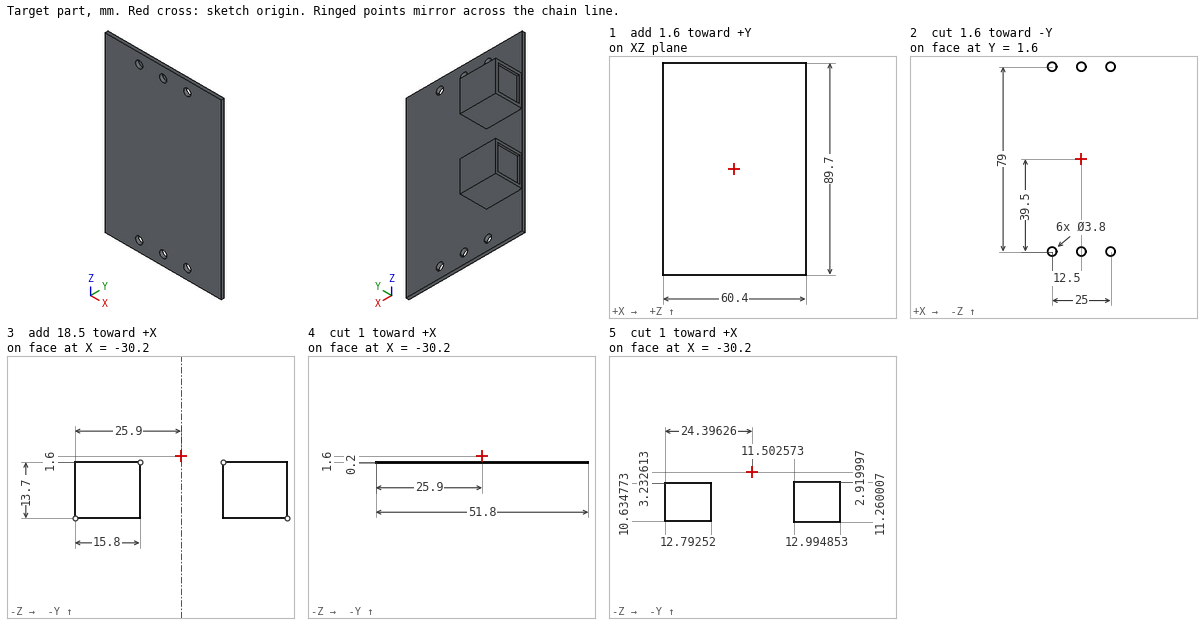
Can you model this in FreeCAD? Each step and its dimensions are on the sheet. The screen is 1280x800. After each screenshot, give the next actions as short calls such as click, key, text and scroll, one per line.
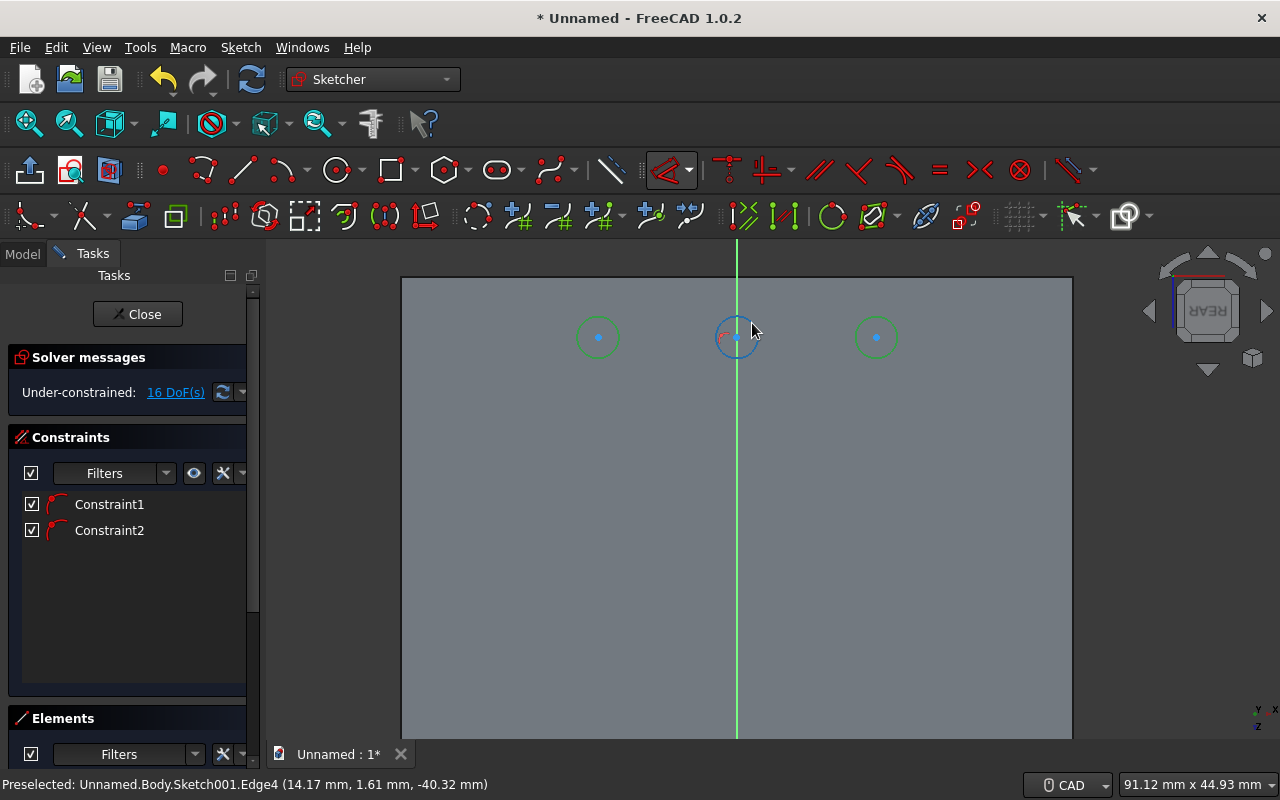
click(752, 323)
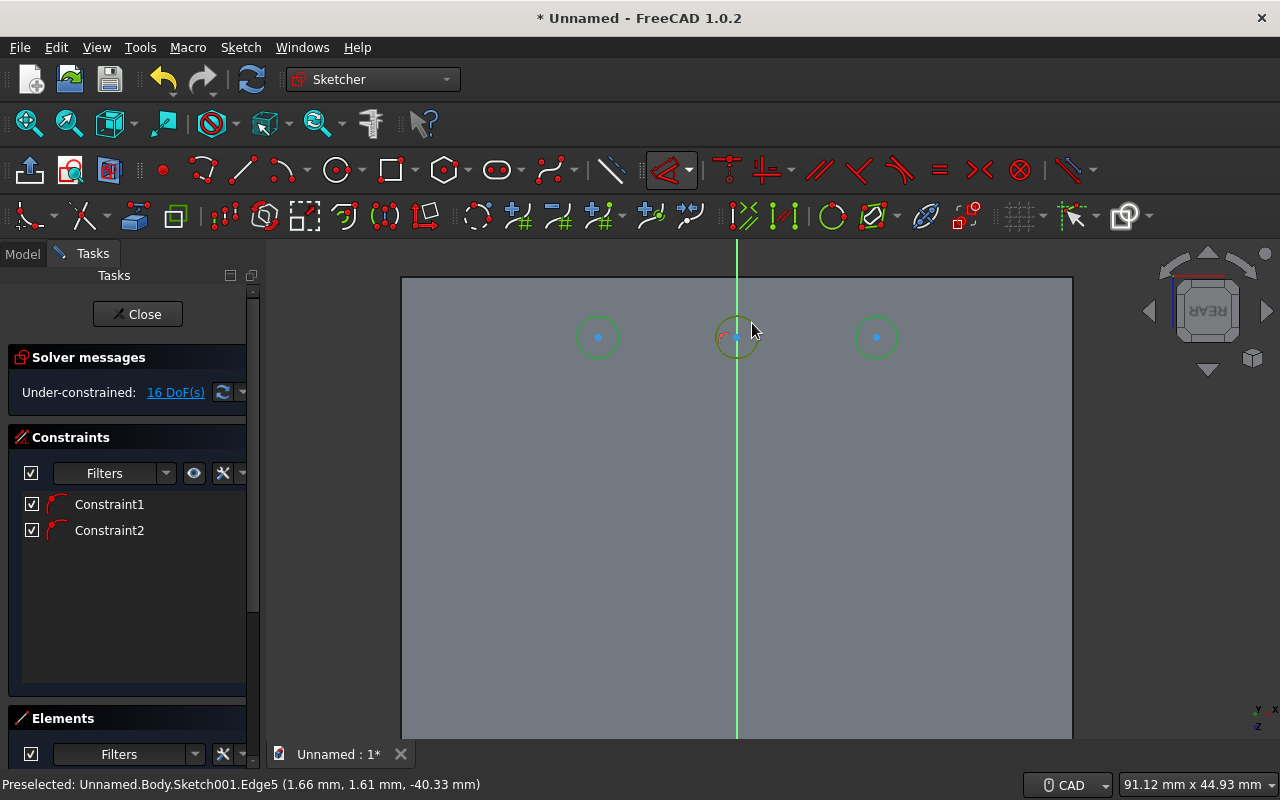
scroll(686, 322, down, 5)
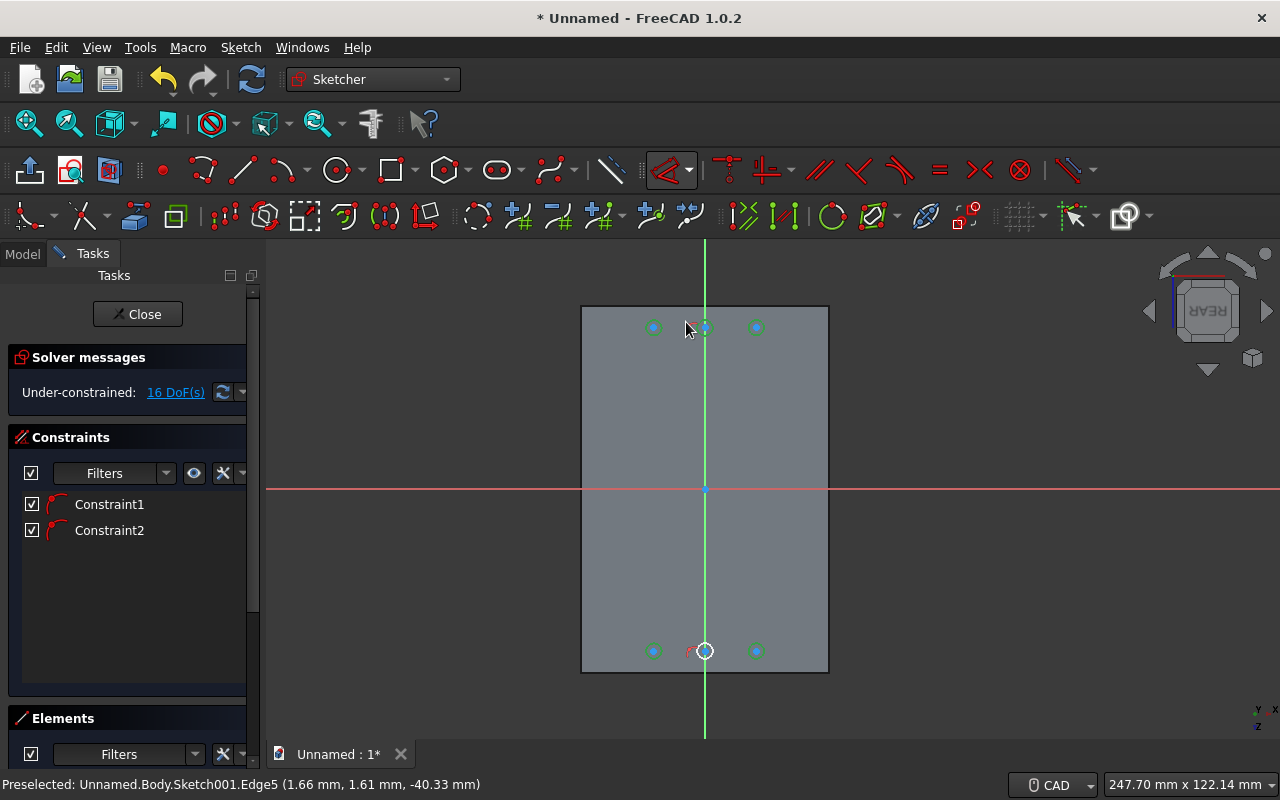
scroll(711, 645, up, 5)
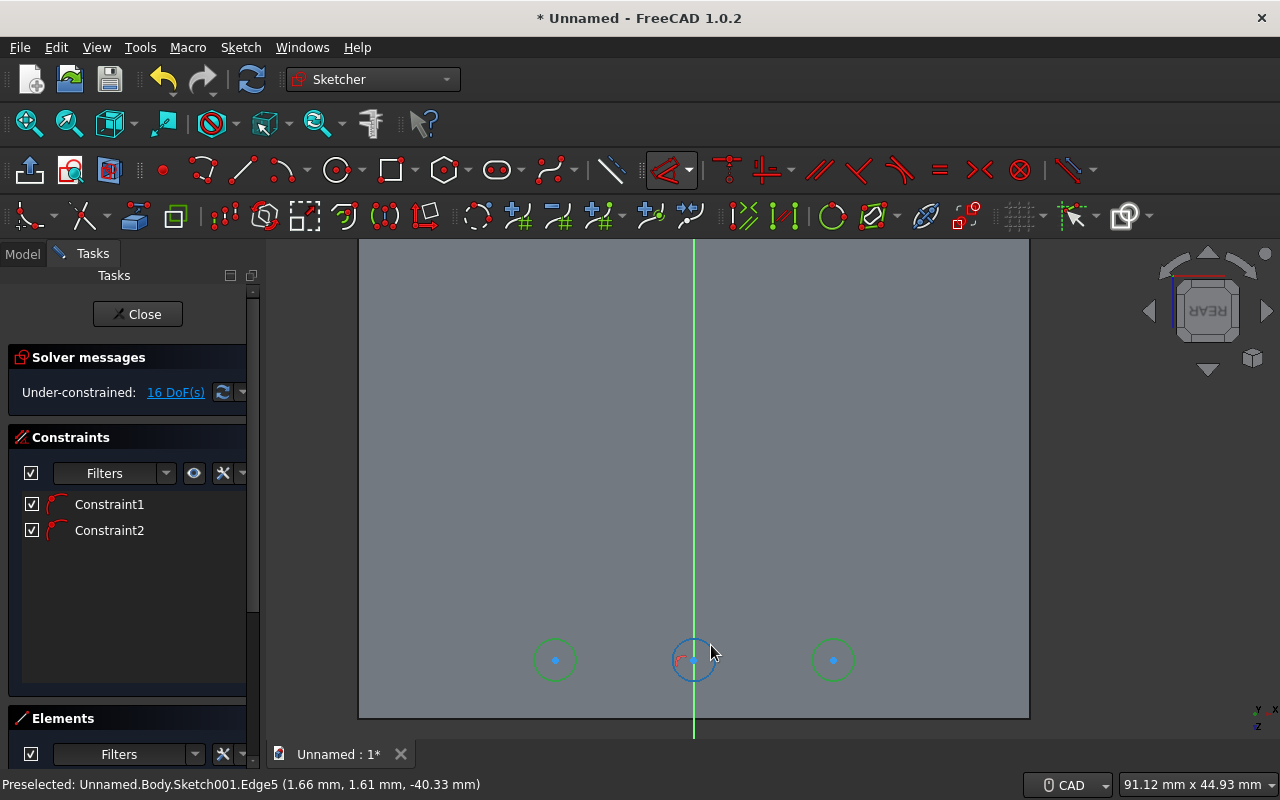
click(709, 645)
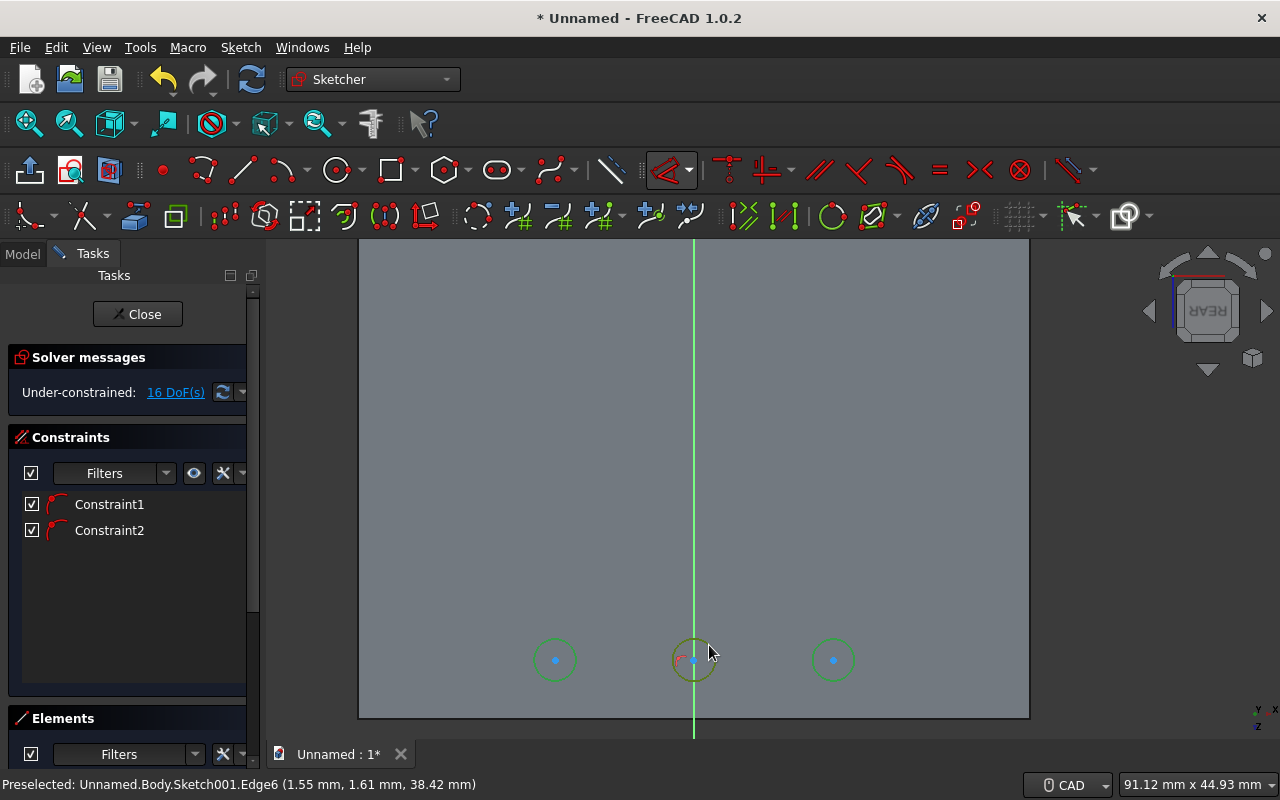
click(940, 170)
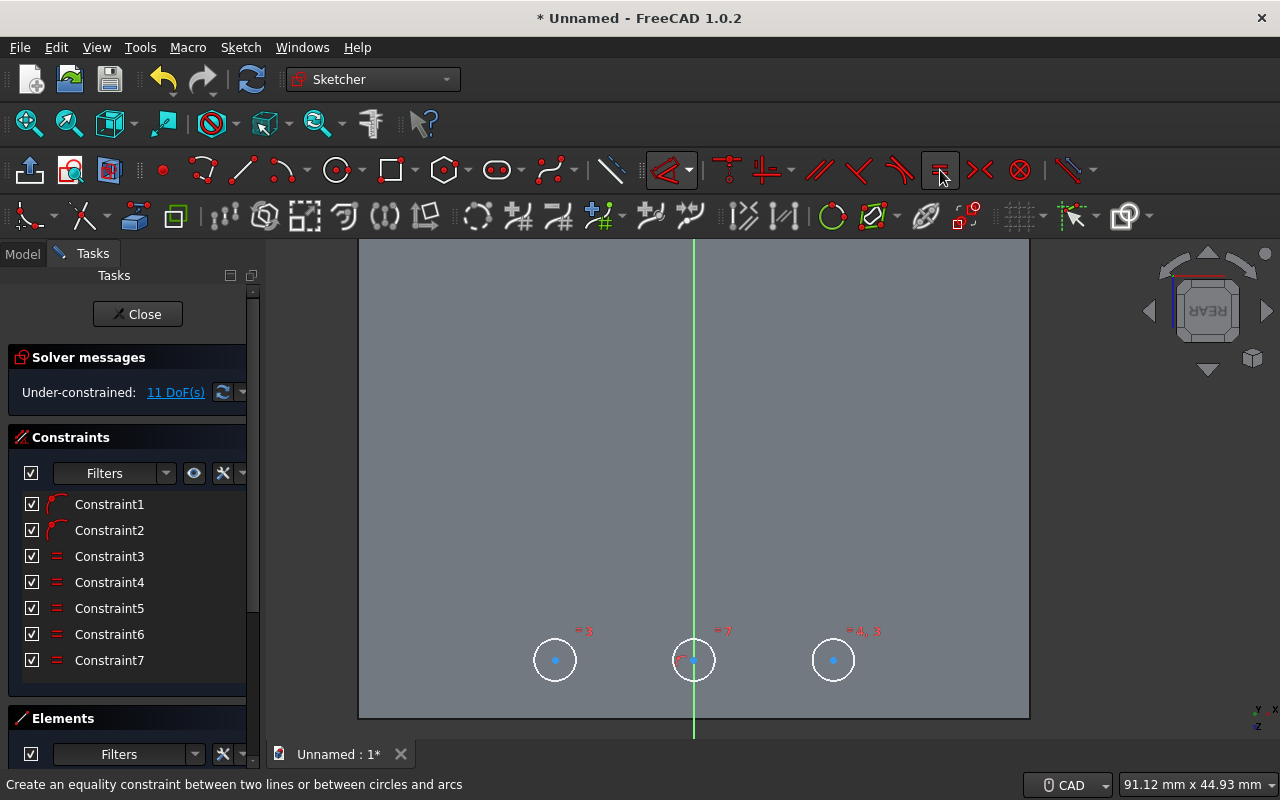
click(555, 660)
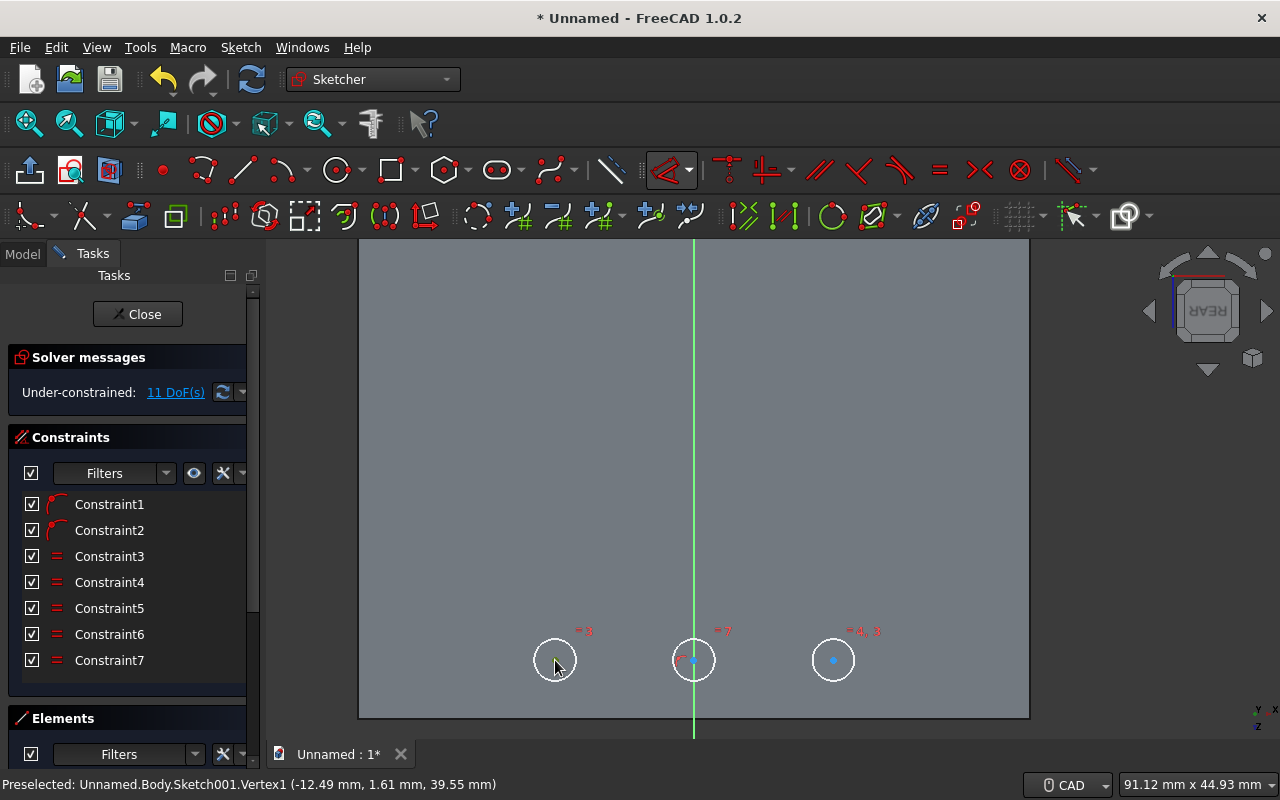
click(833, 660)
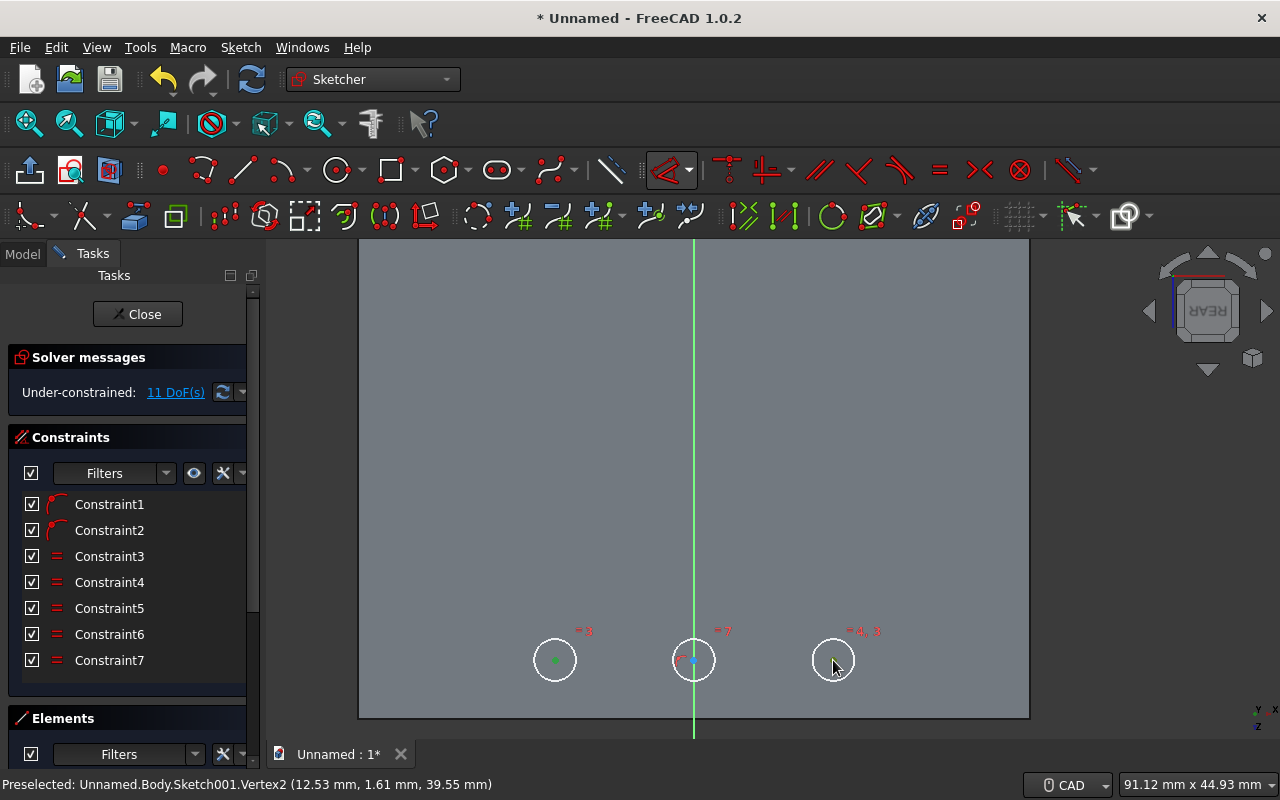
click(794, 170)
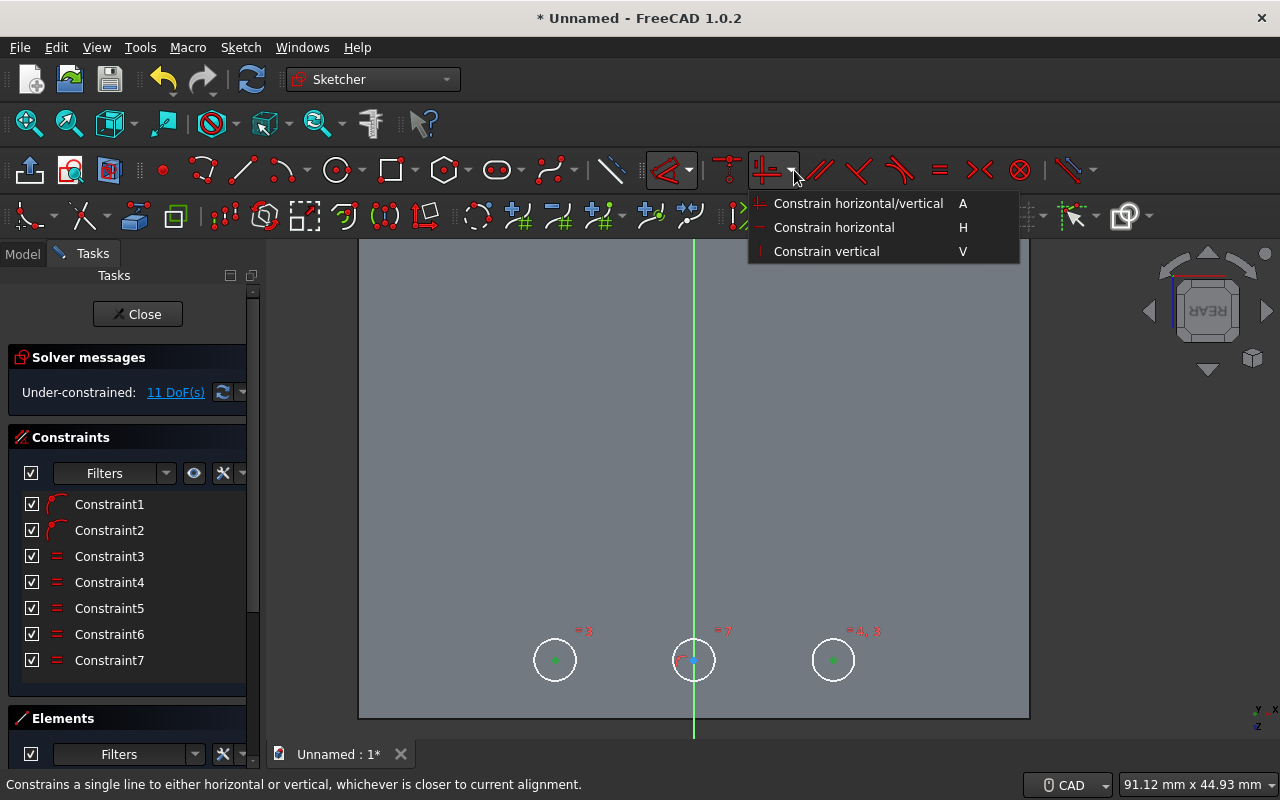
click(884, 227)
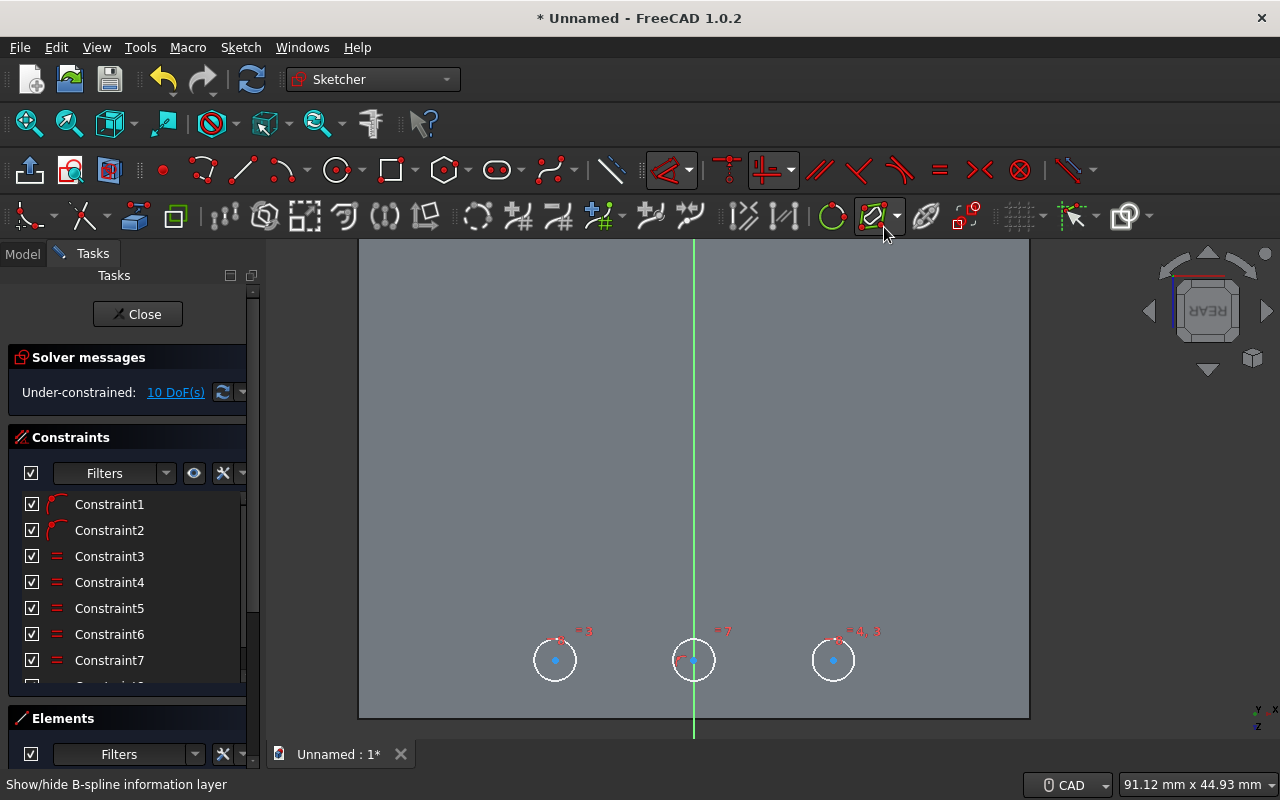
click(555, 660)